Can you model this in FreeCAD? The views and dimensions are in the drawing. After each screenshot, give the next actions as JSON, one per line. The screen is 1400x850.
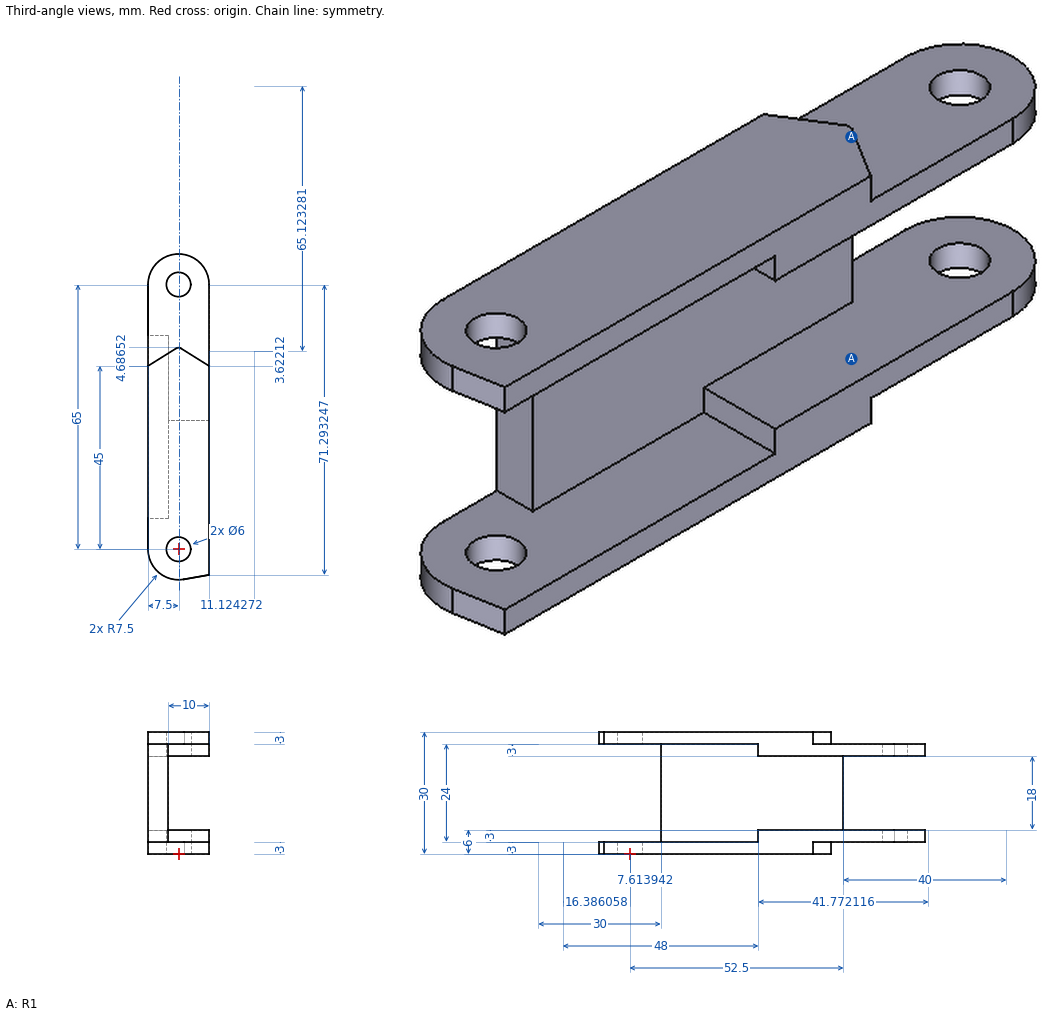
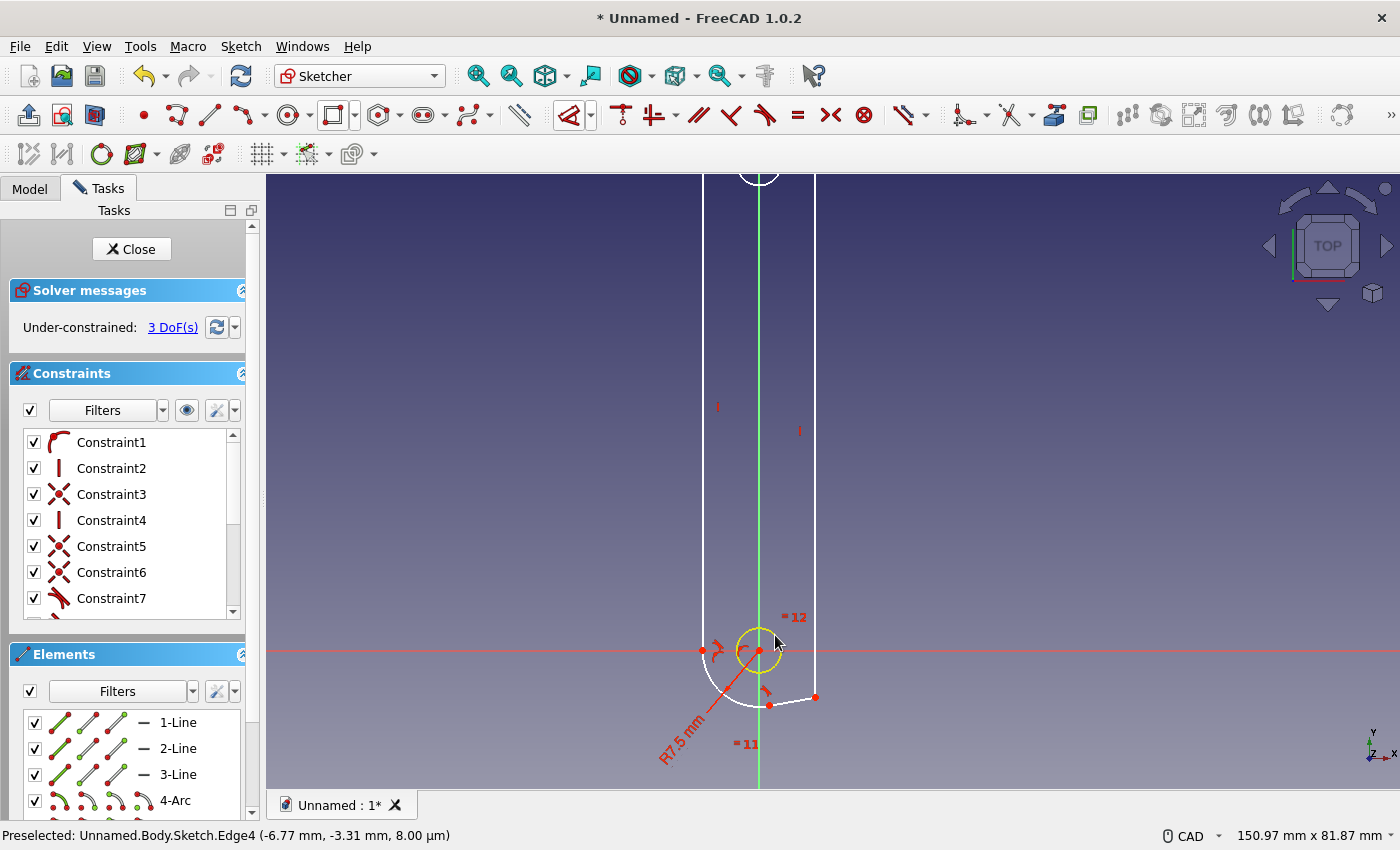
{"action": "left_click", "coordinate": [775, 635]}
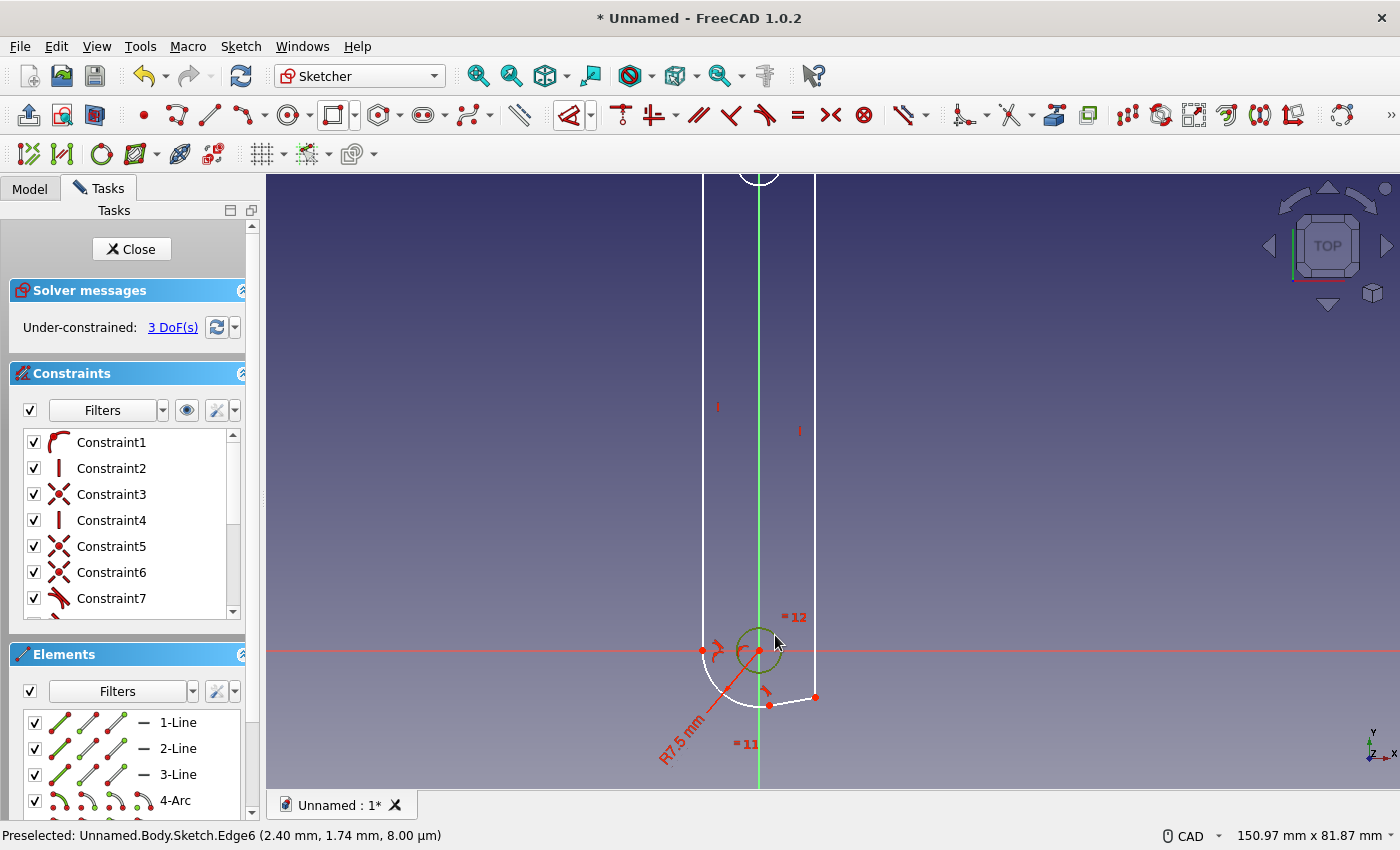
{"action": "key", "text": "k o"}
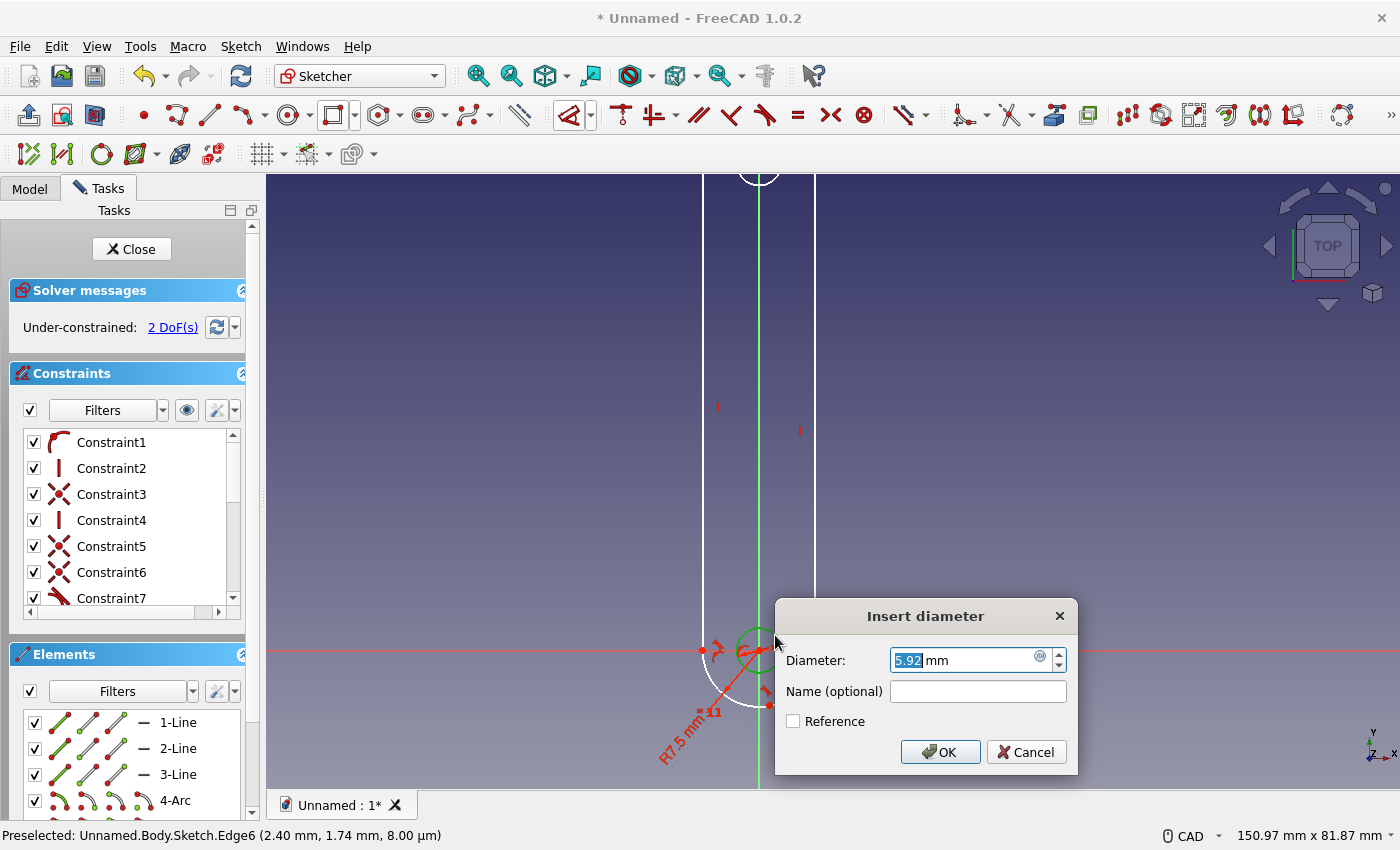
{"action": "type", "text": "6"}
{"action": "key", "text": "Return"}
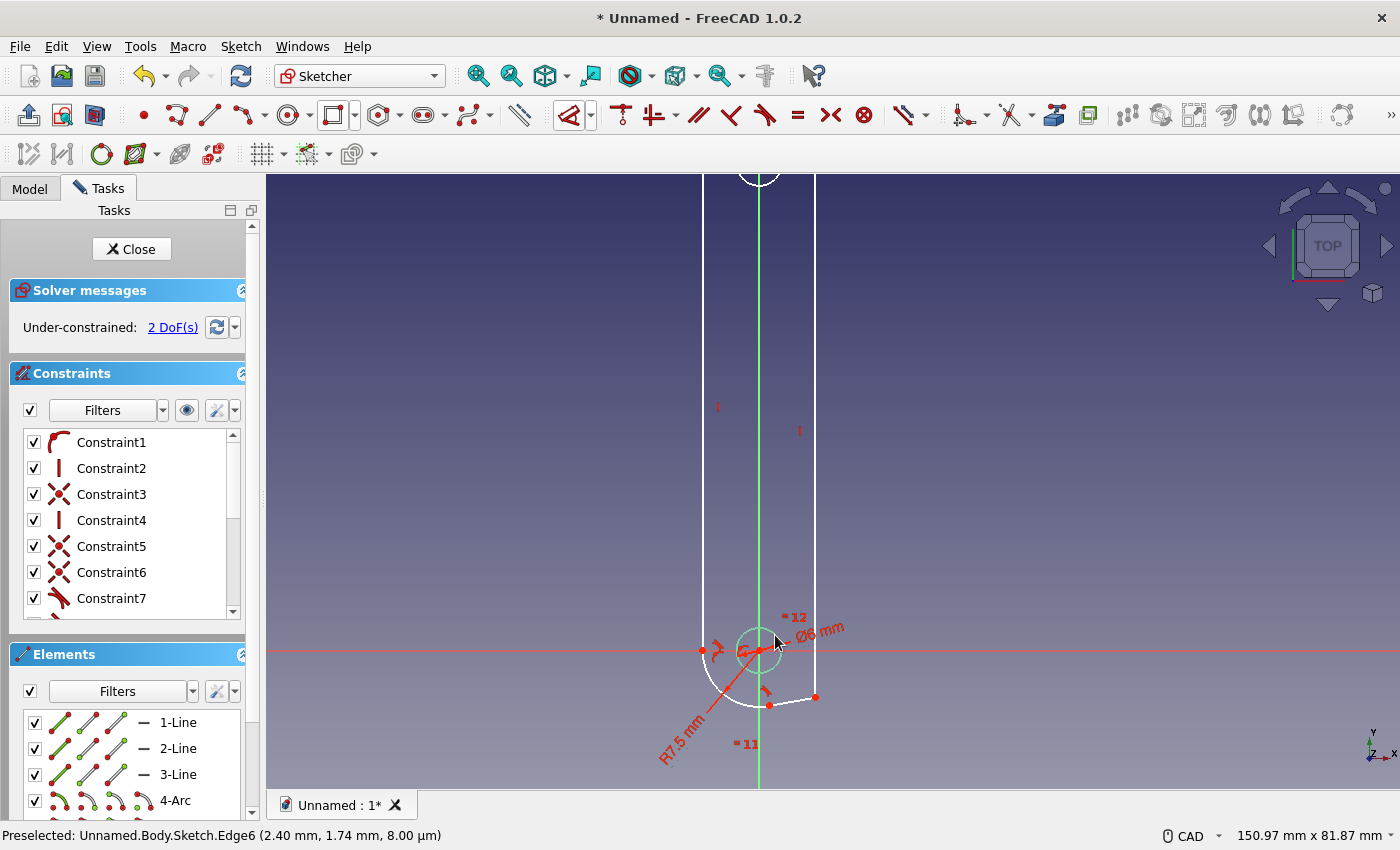
{"action": "left_click", "coordinate": [703, 309]}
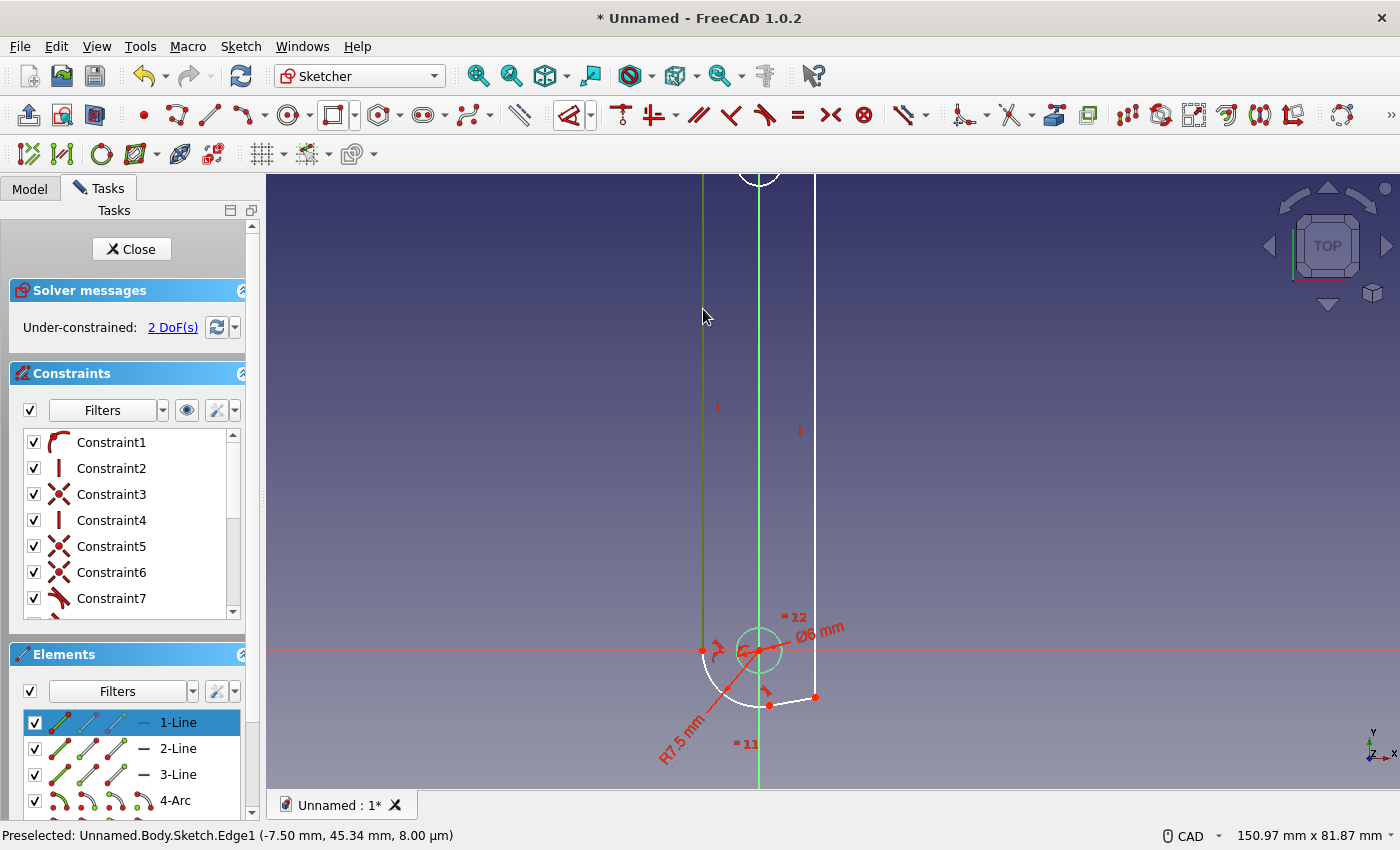
{"action": "key", "text": "i"}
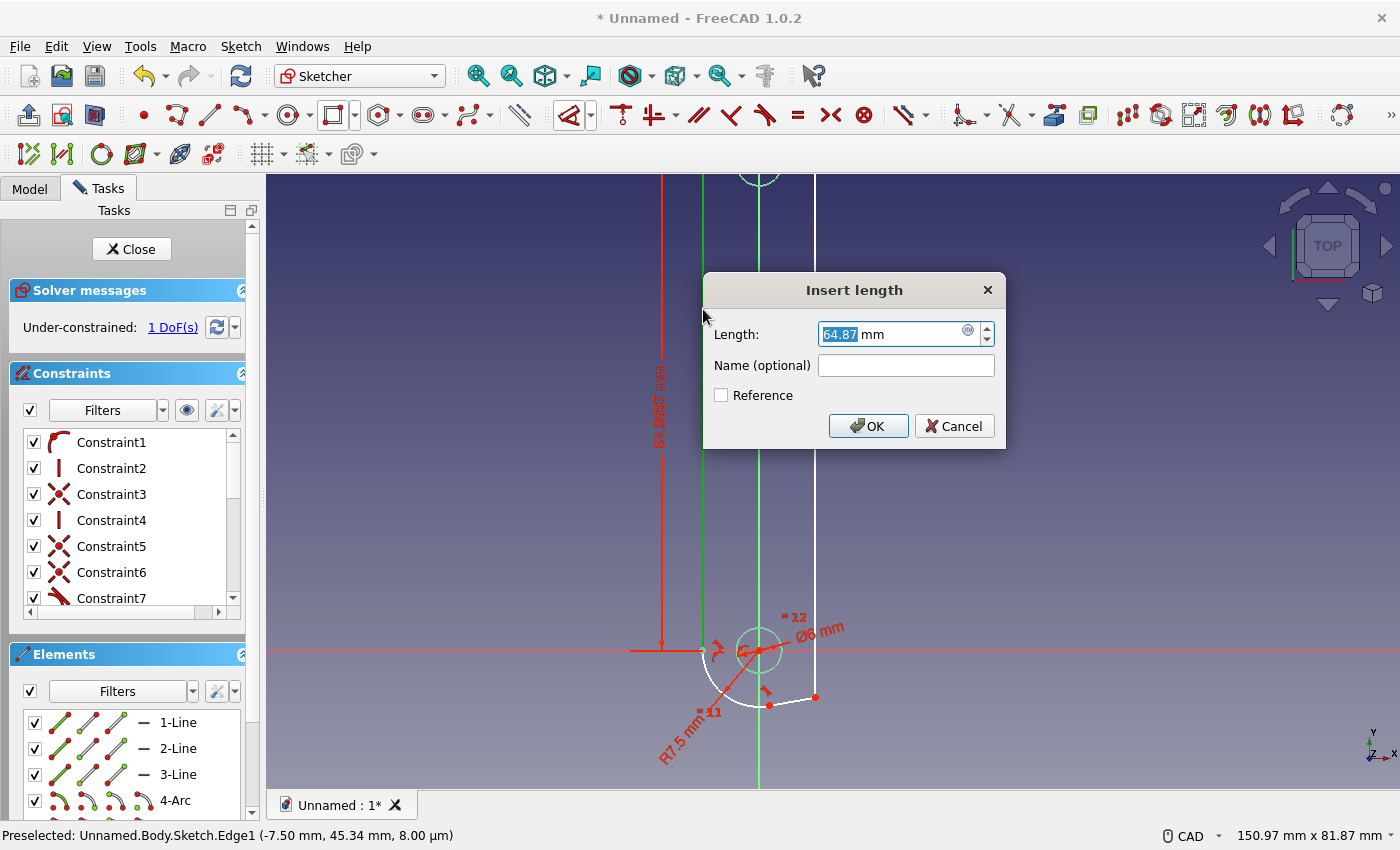
{"action": "type", "text": "65"}
{"action": "key", "text": "Return"}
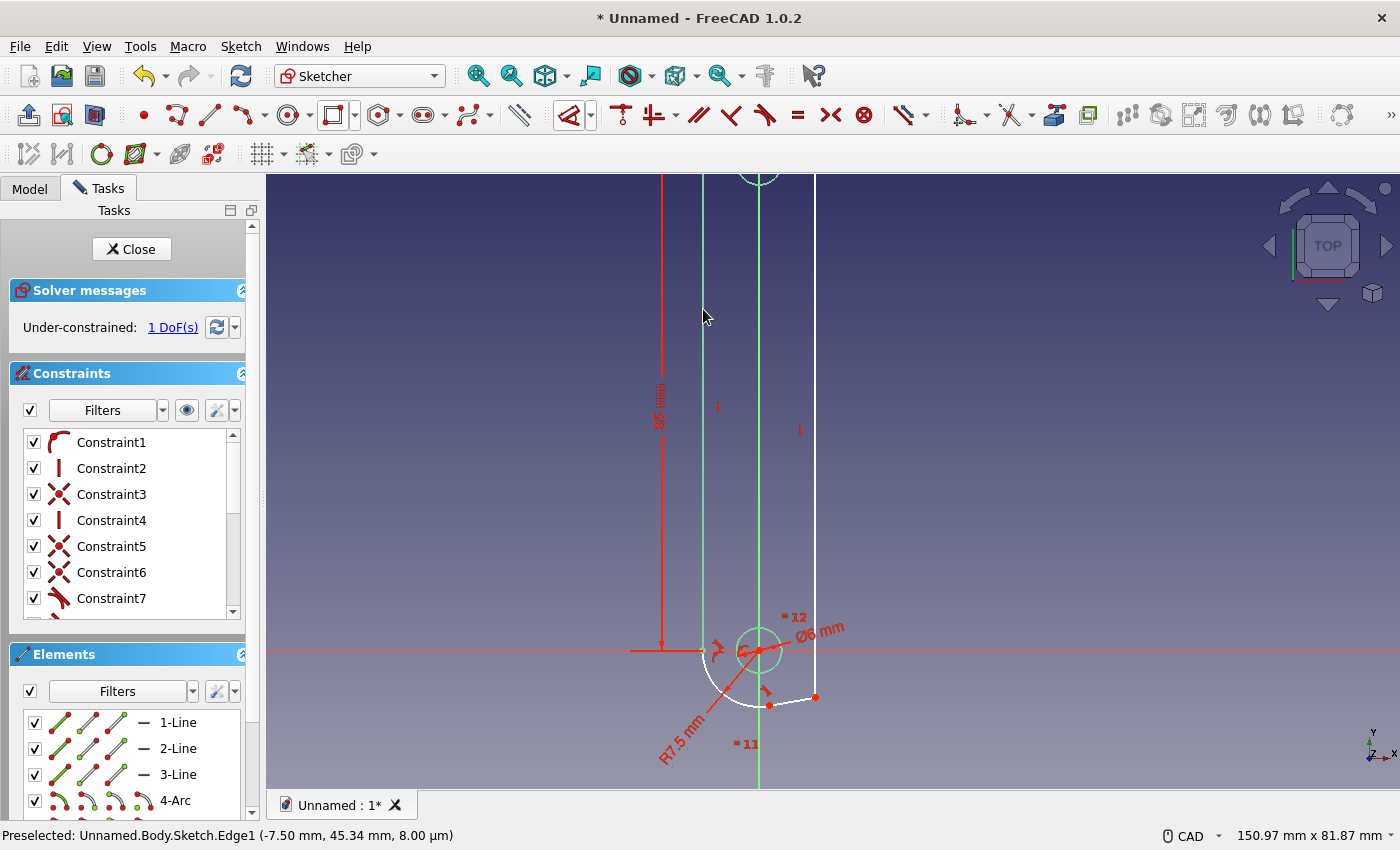
{"action": "left_click", "coordinate": [815, 537]}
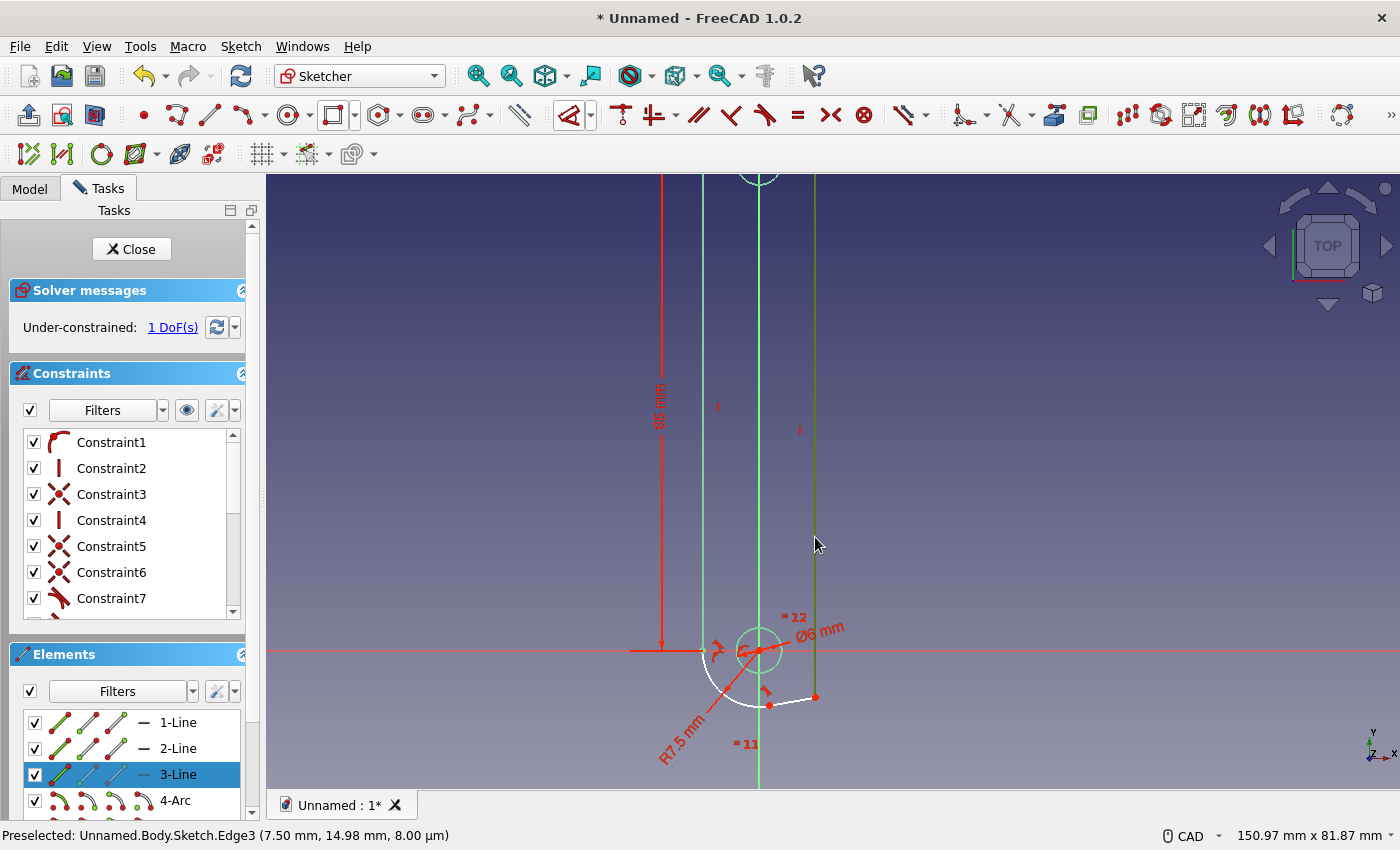
{"action": "key", "text": "i"}